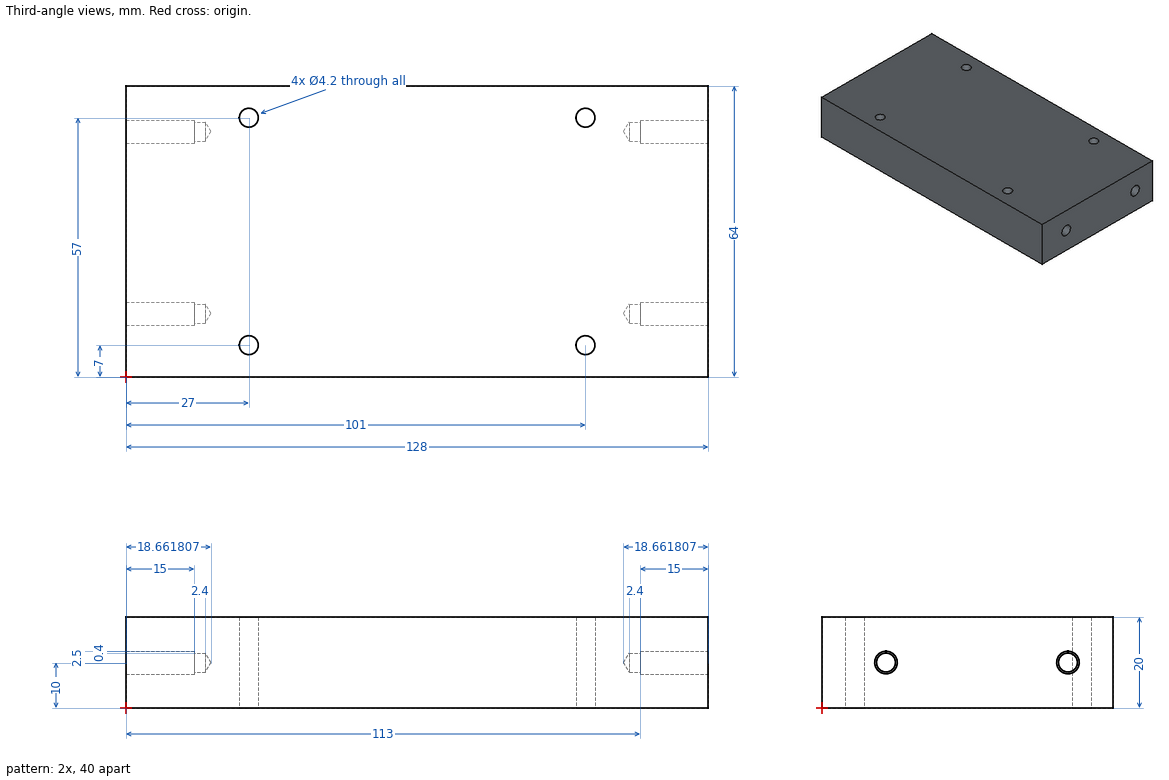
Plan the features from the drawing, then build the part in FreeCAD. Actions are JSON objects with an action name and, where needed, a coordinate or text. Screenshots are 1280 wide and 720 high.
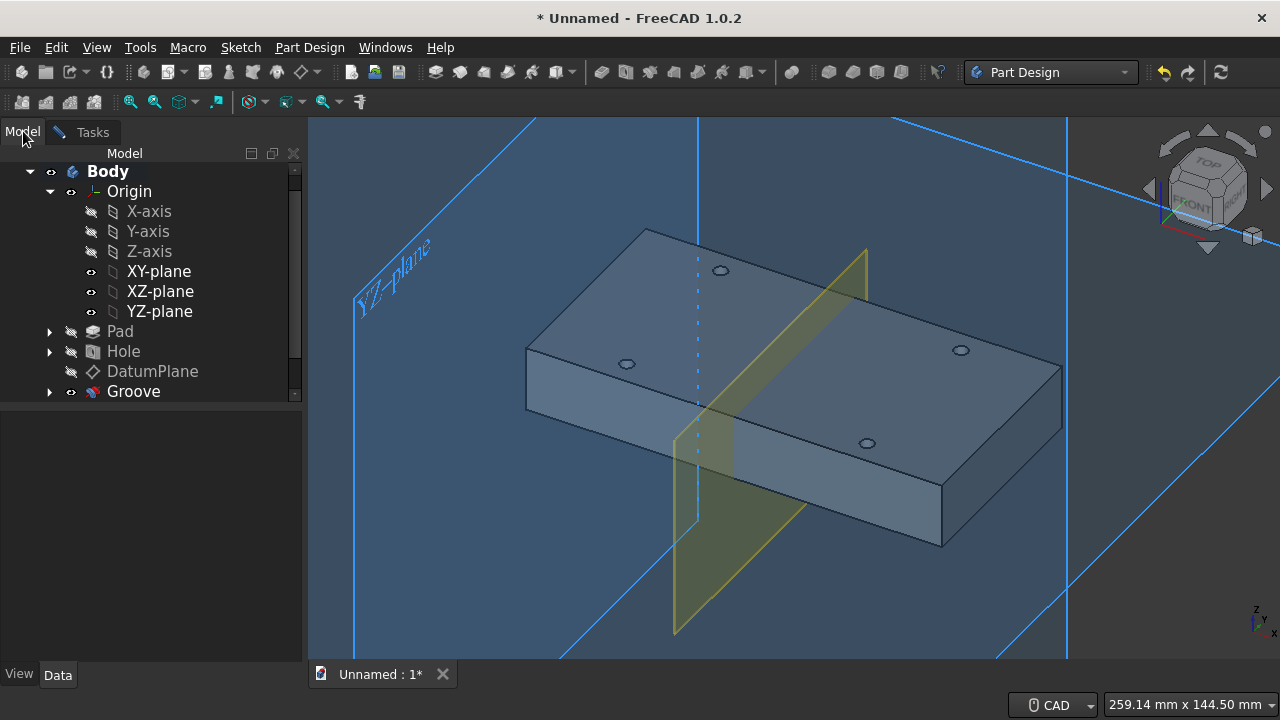
{"action": "scroll", "coordinate": [120, 287], "scroll_direction": "down", "scroll_amount": 3}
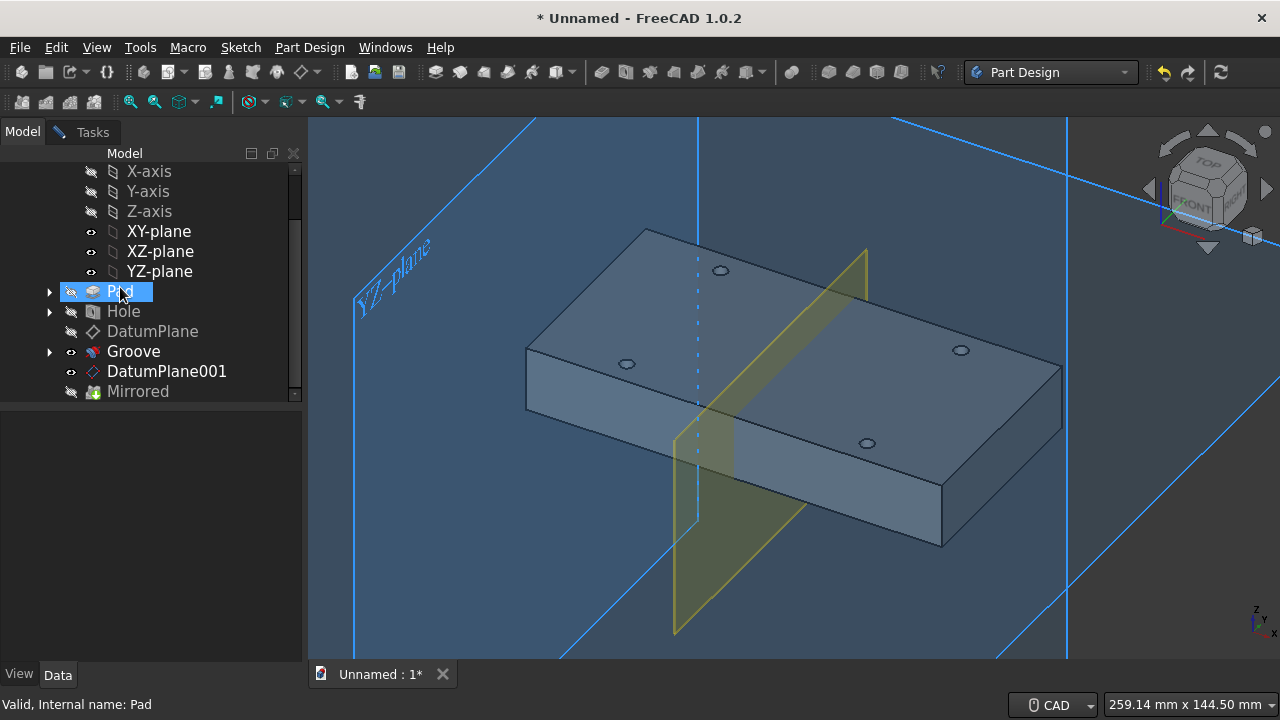
{"action": "left_click", "coordinate": [116, 372]}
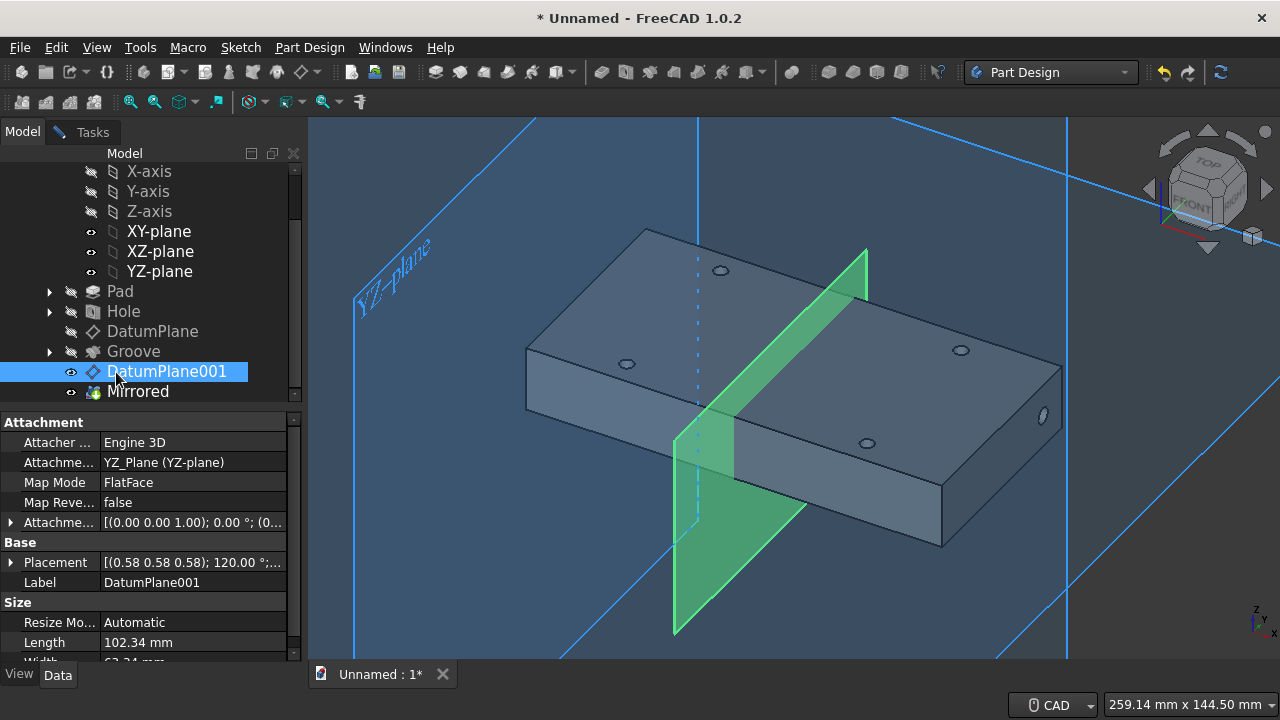
{"action": "left_click", "coordinate": [84, 131]}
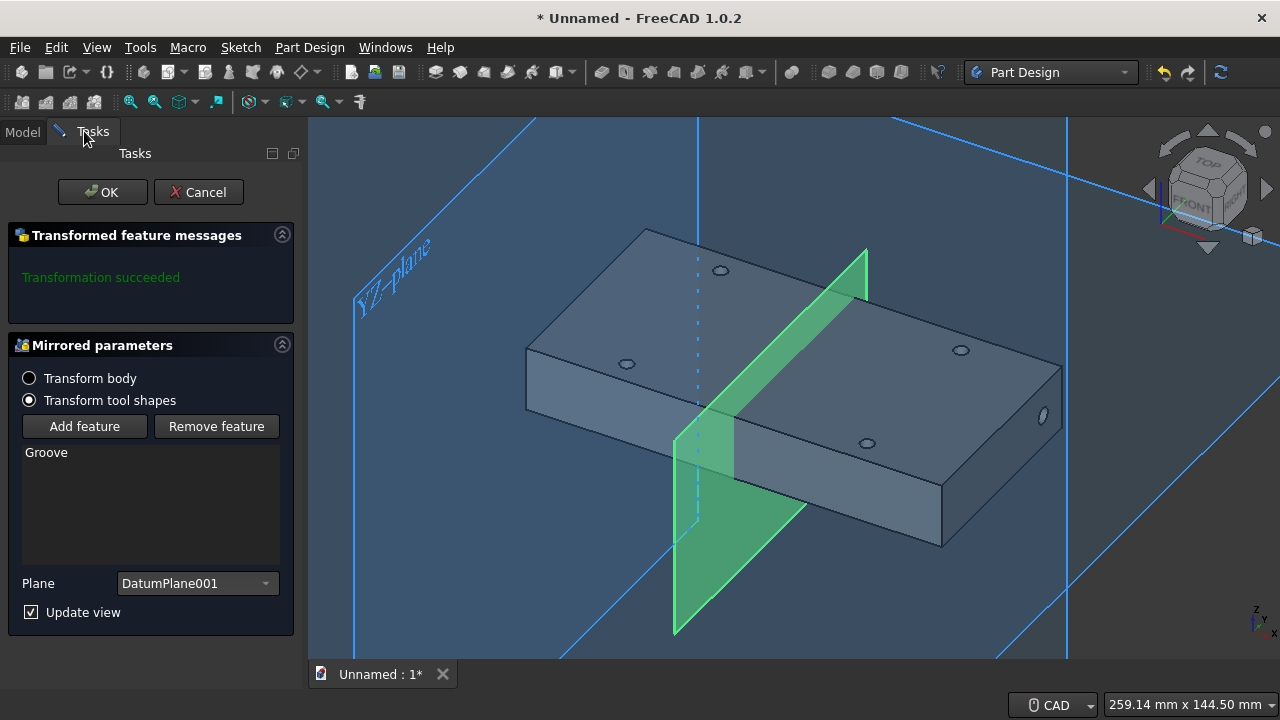
{"action": "left_click", "coordinate": [103, 192]}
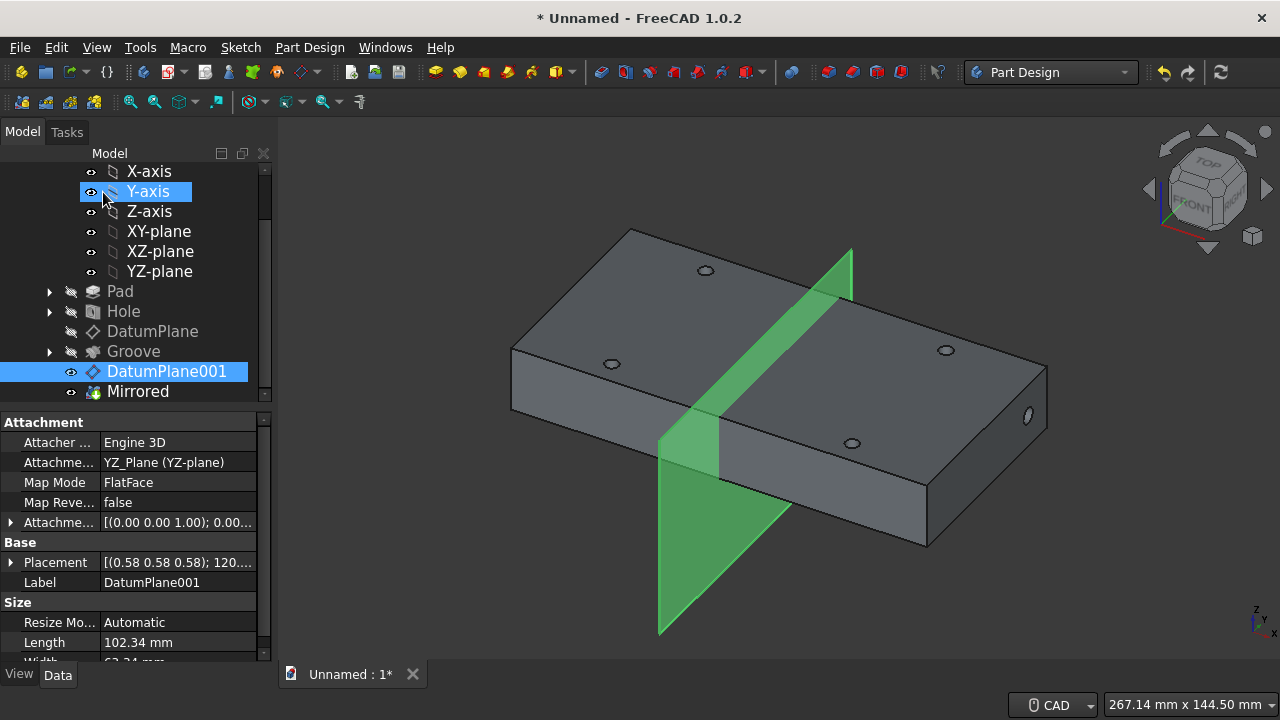
{"action": "left_click", "coordinate": [116, 372]}
{"action": "key", "text": "space"}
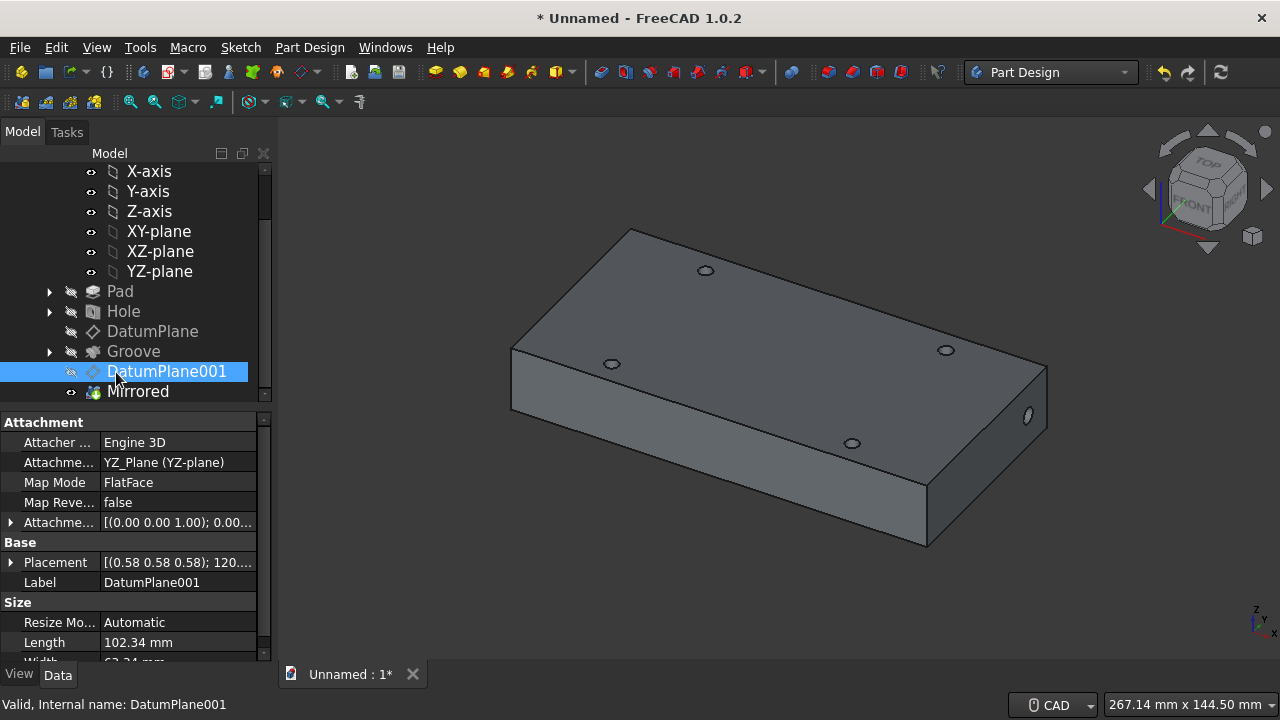
{"action": "left_click", "coordinate": [116, 352]}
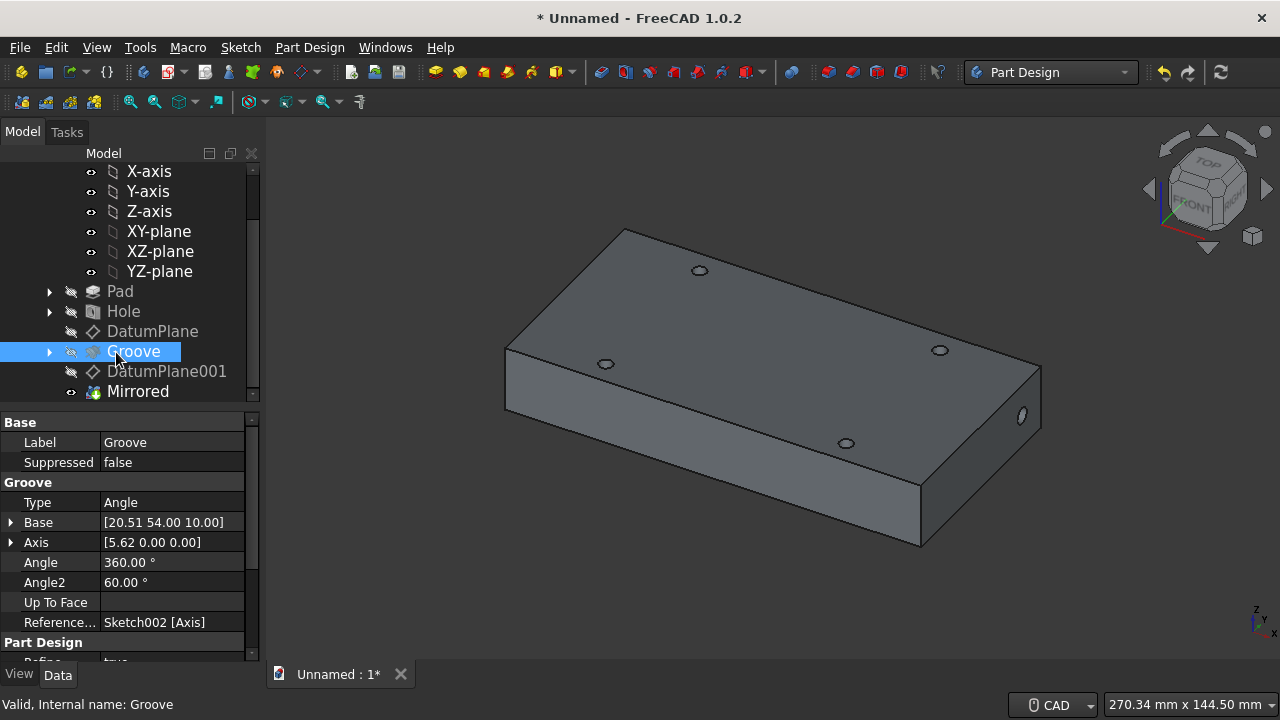
{"action": "left_click", "coordinate": [46, 102]}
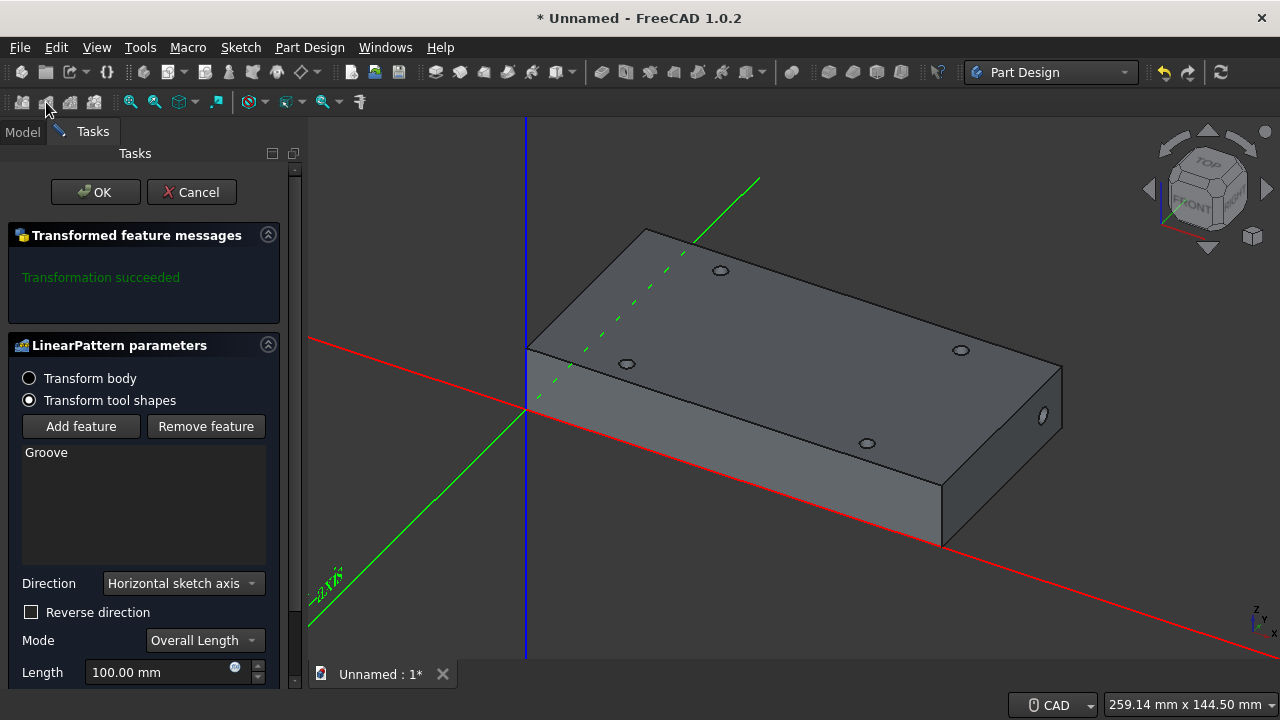
{"action": "left_click", "coordinate": [184, 584]}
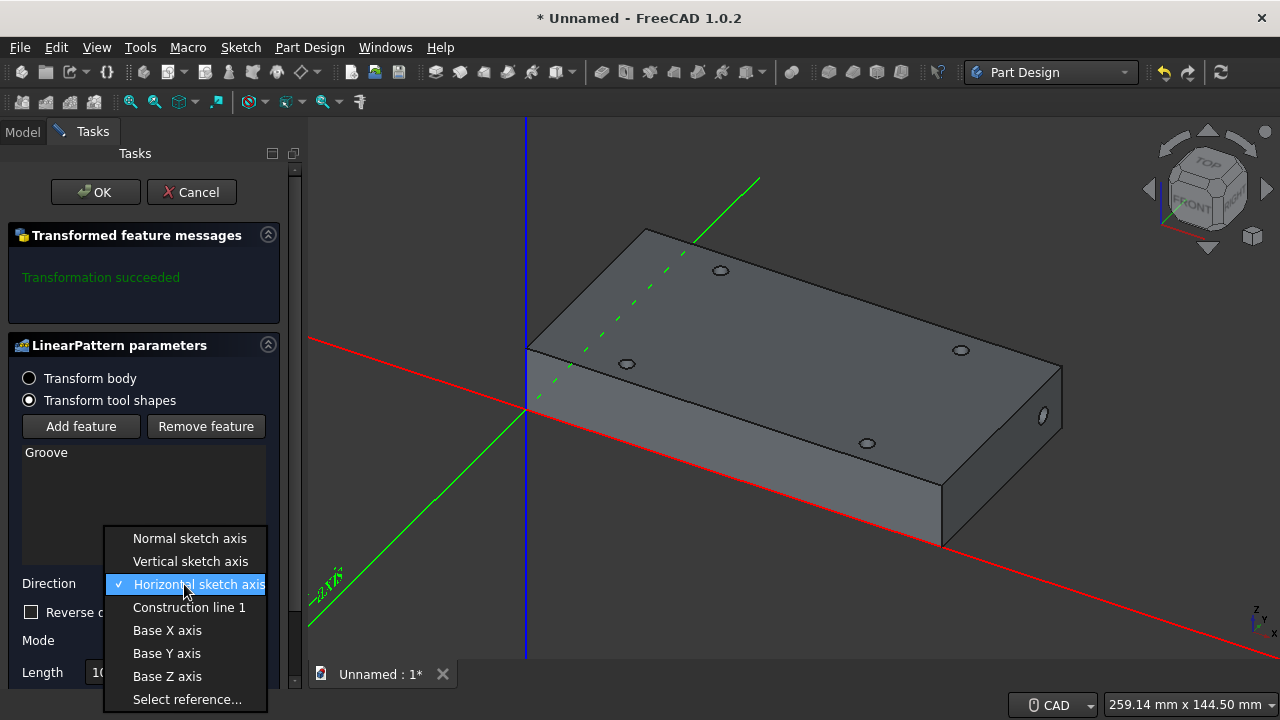
{"action": "left_click", "coordinate": [184, 654]}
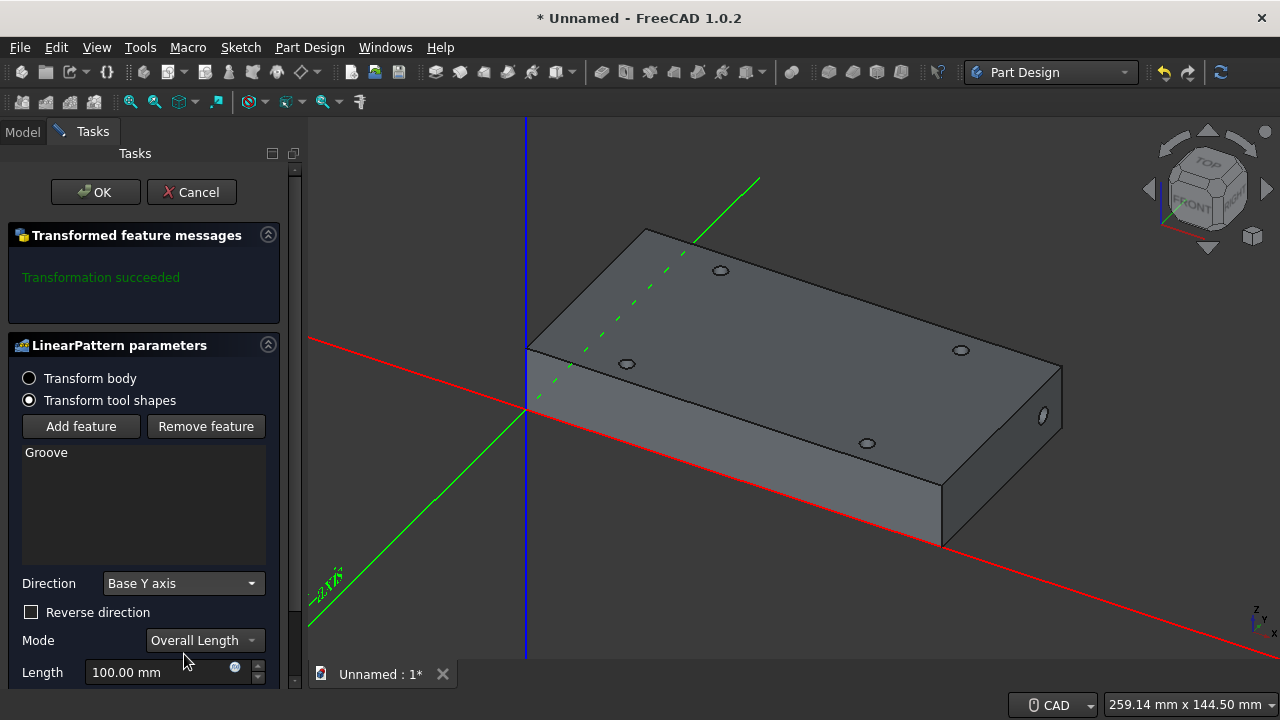
{"action": "left_click", "coordinate": [206, 640]}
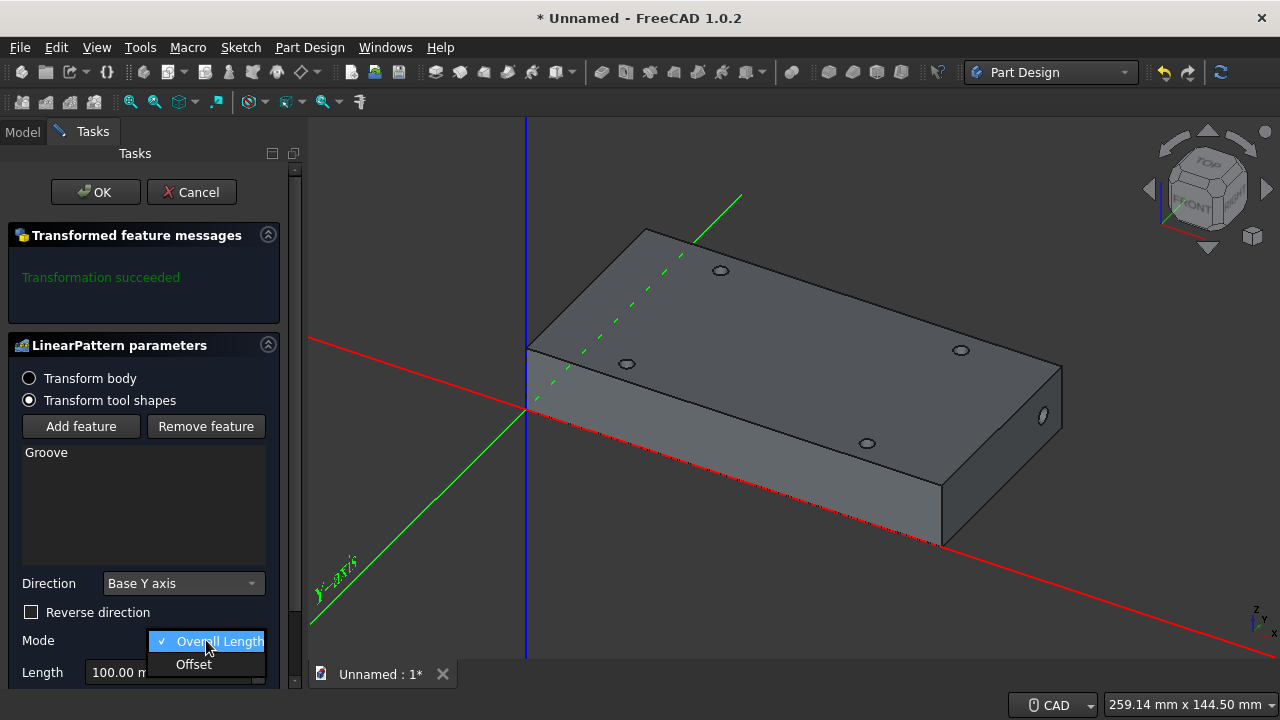
{"action": "left_click", "coordinate": [206, 664]}